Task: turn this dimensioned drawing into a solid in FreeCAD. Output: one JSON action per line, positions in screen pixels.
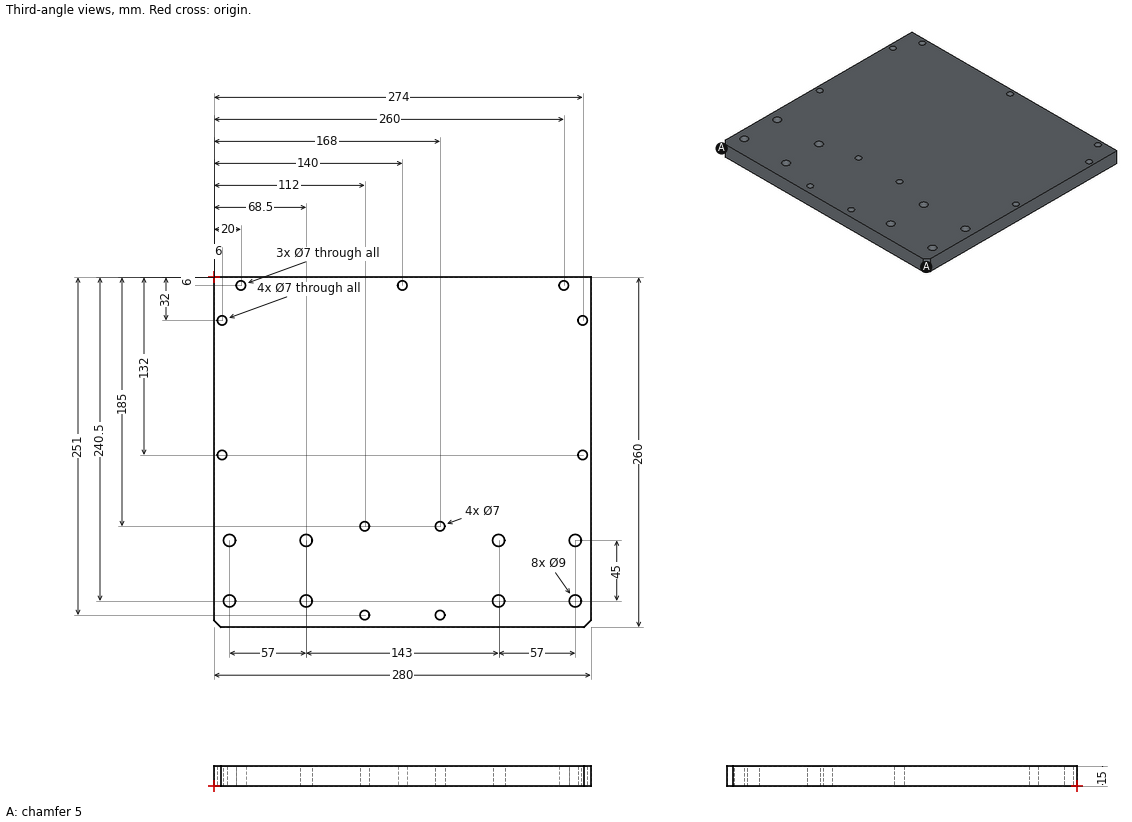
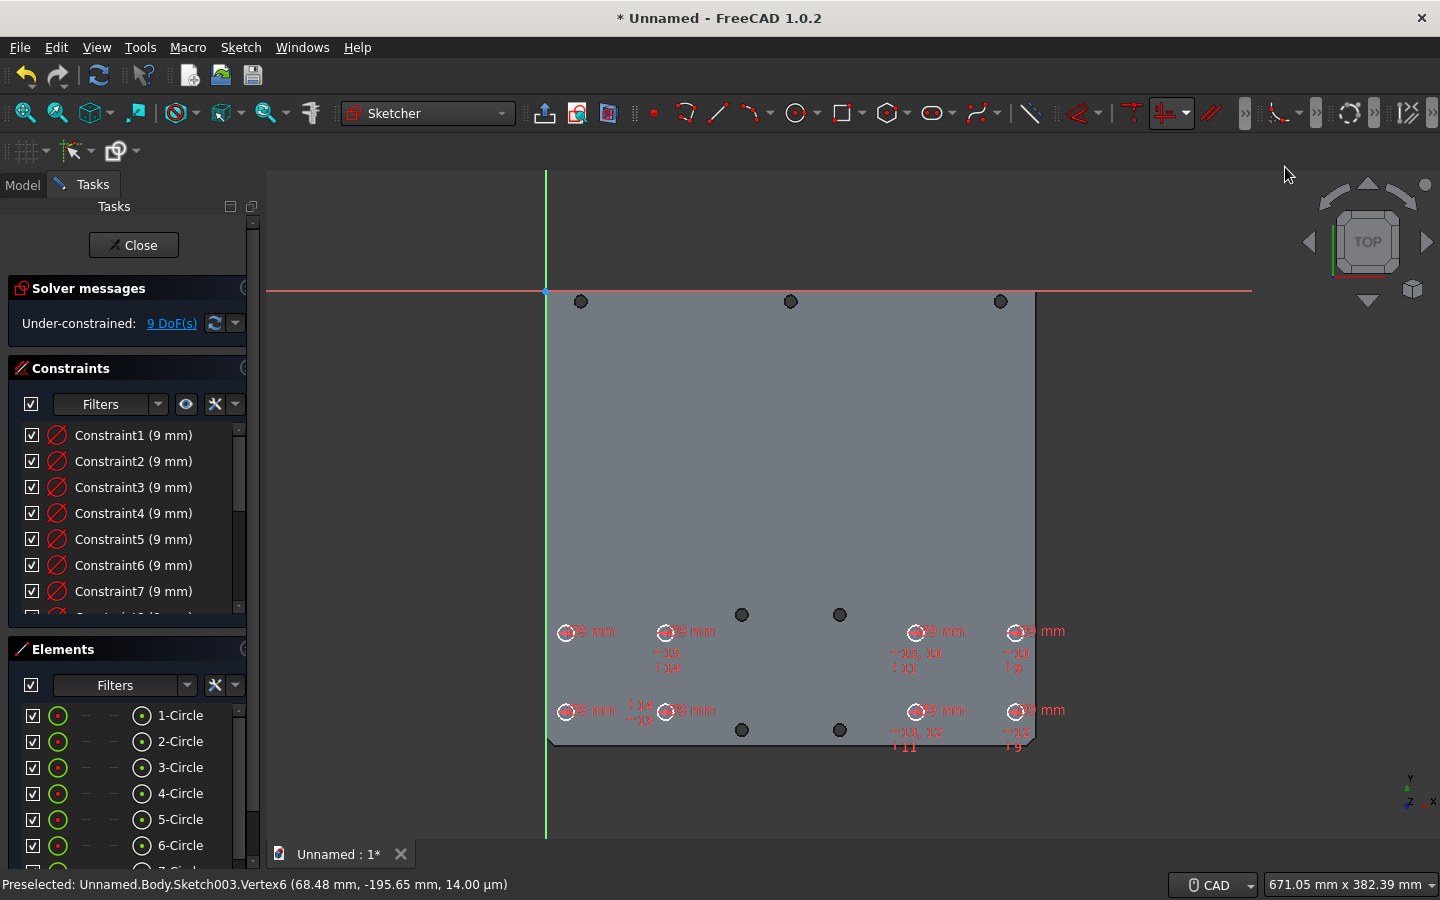
{"action": "left_click", "coordinate": [666, 633]}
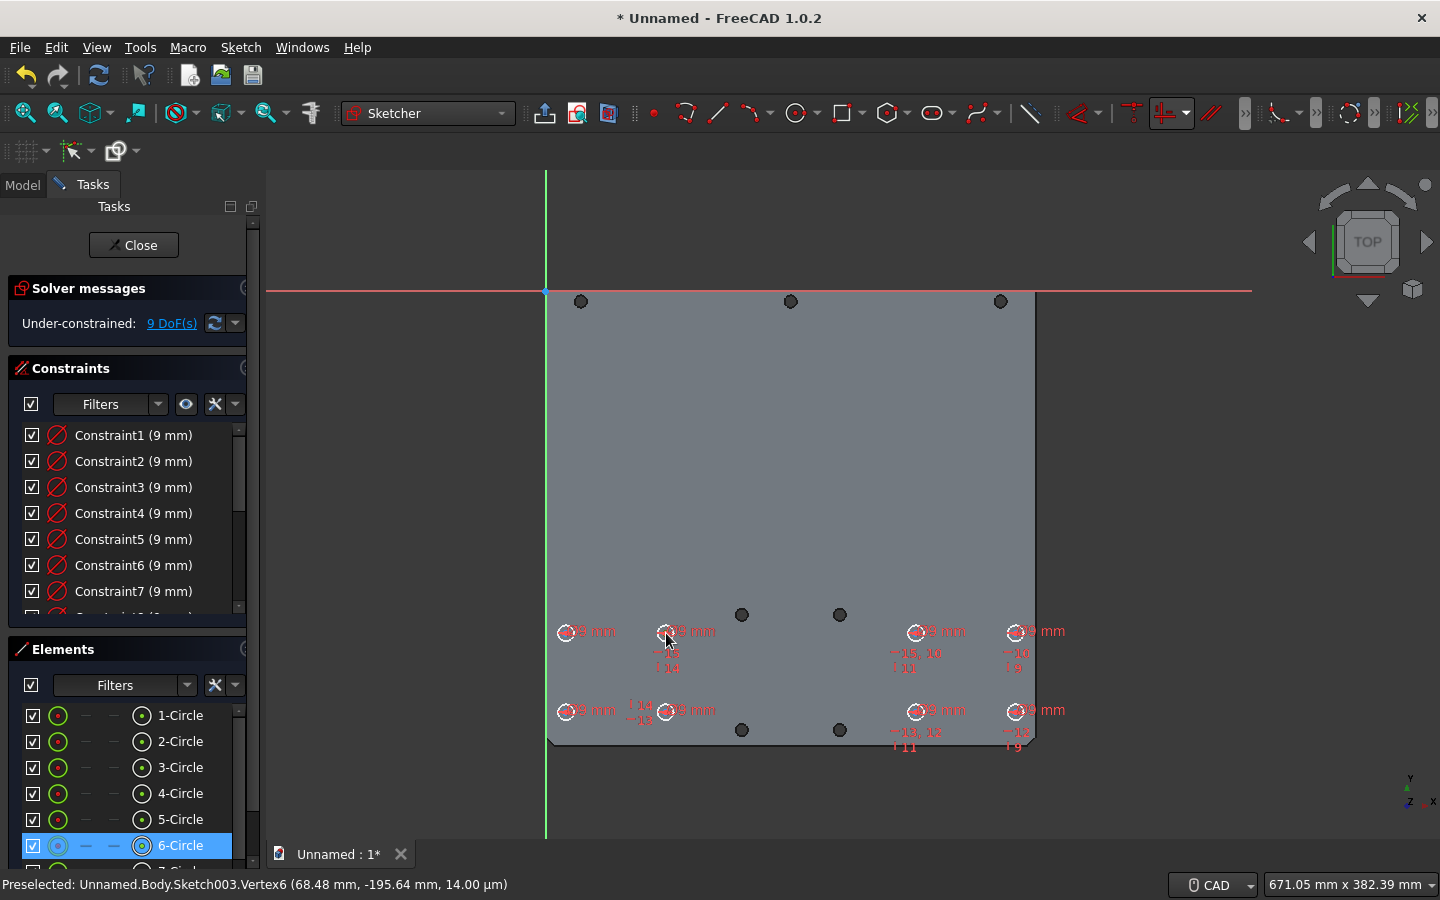
{"action": "left_click", "coordinate": [566, 633]}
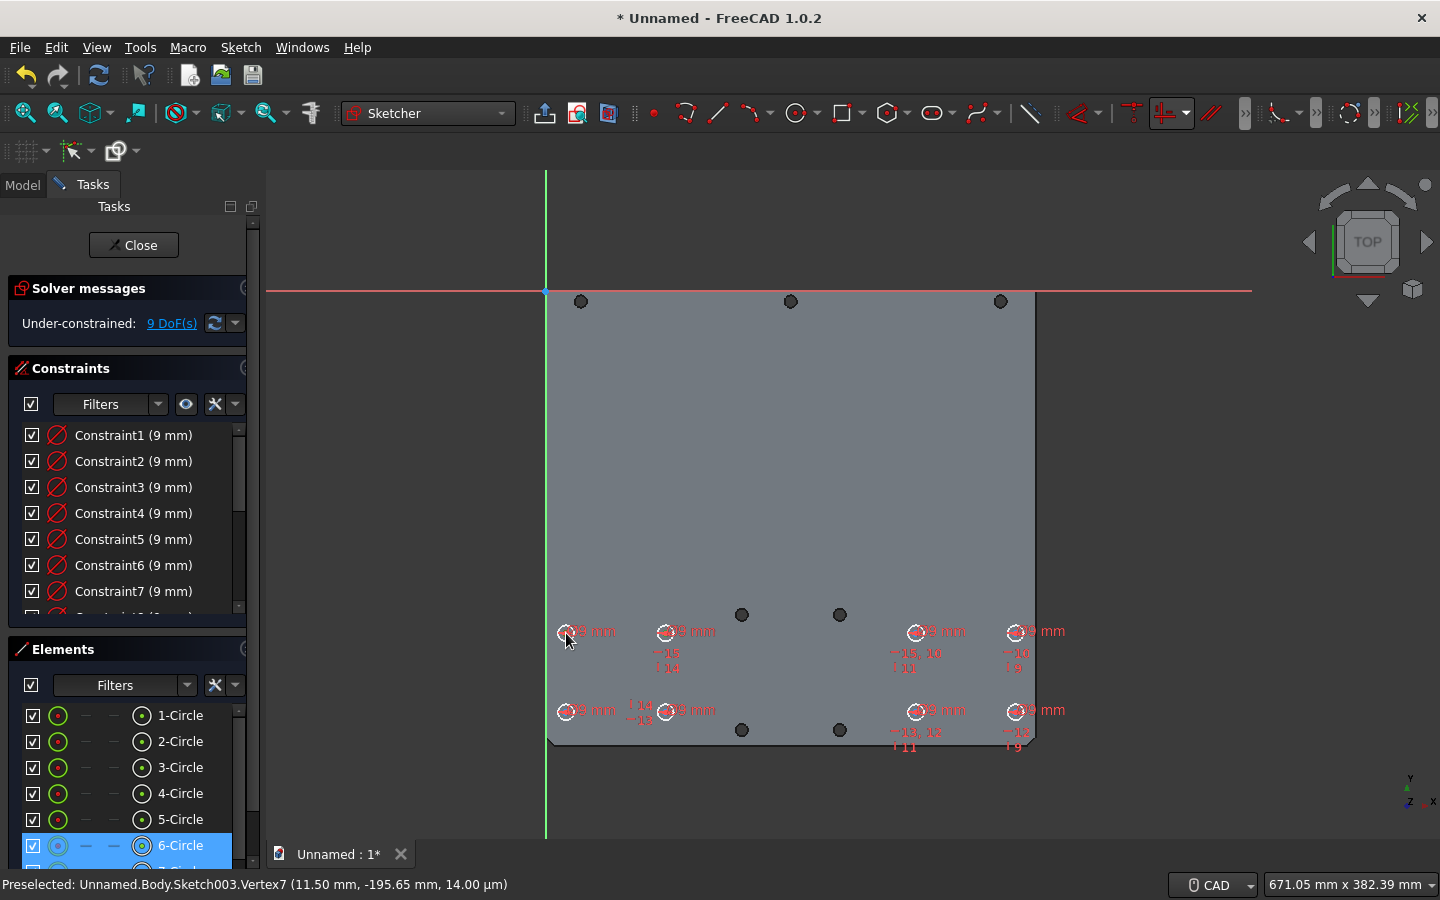
{"action": "key", "text": "h"}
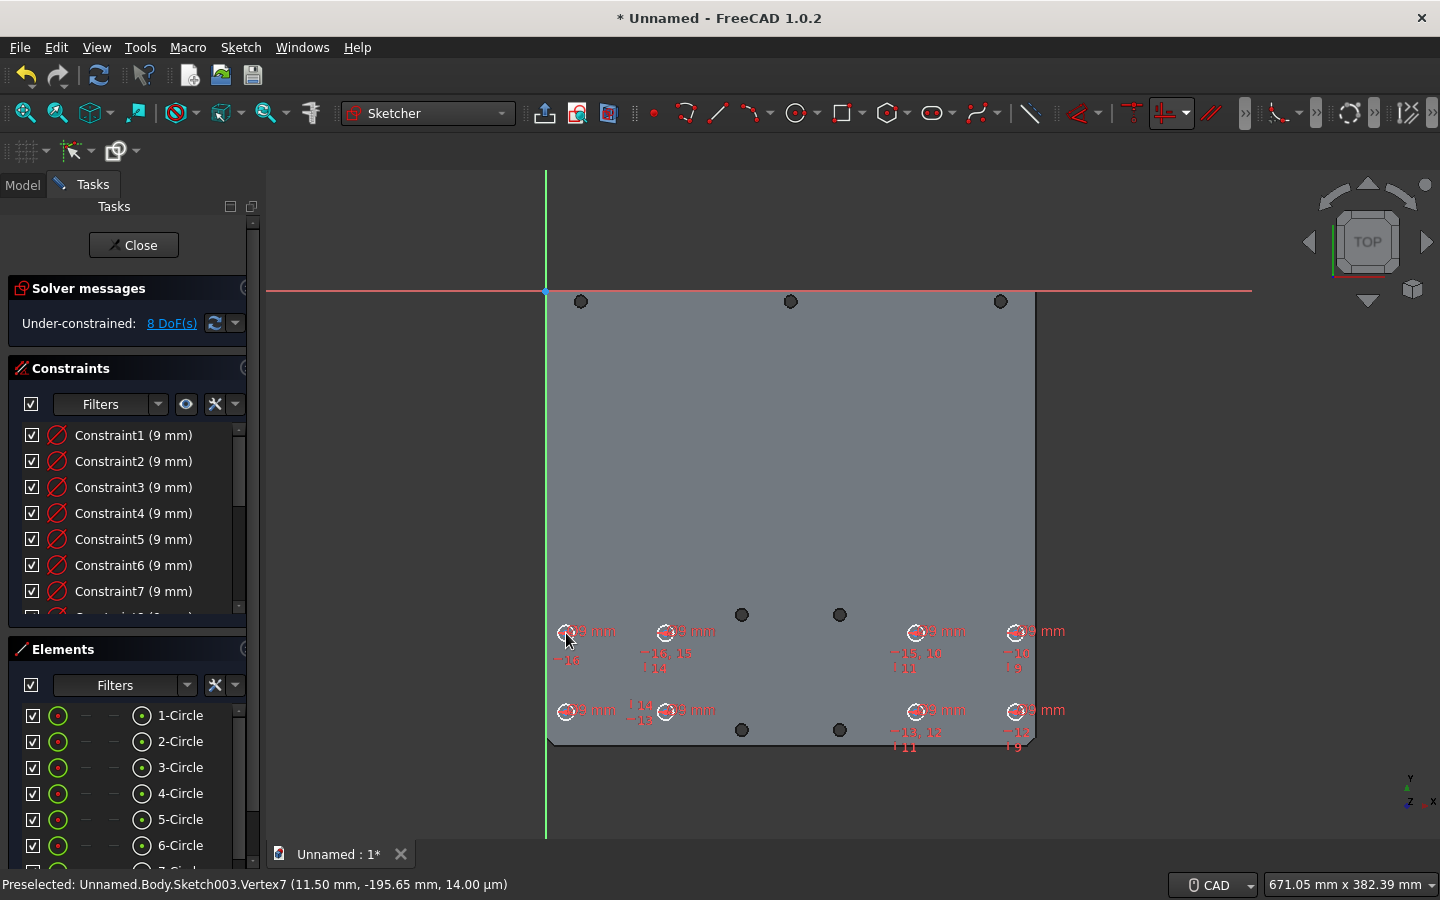
{"action": "left_click", "coordinate": [566, 633]}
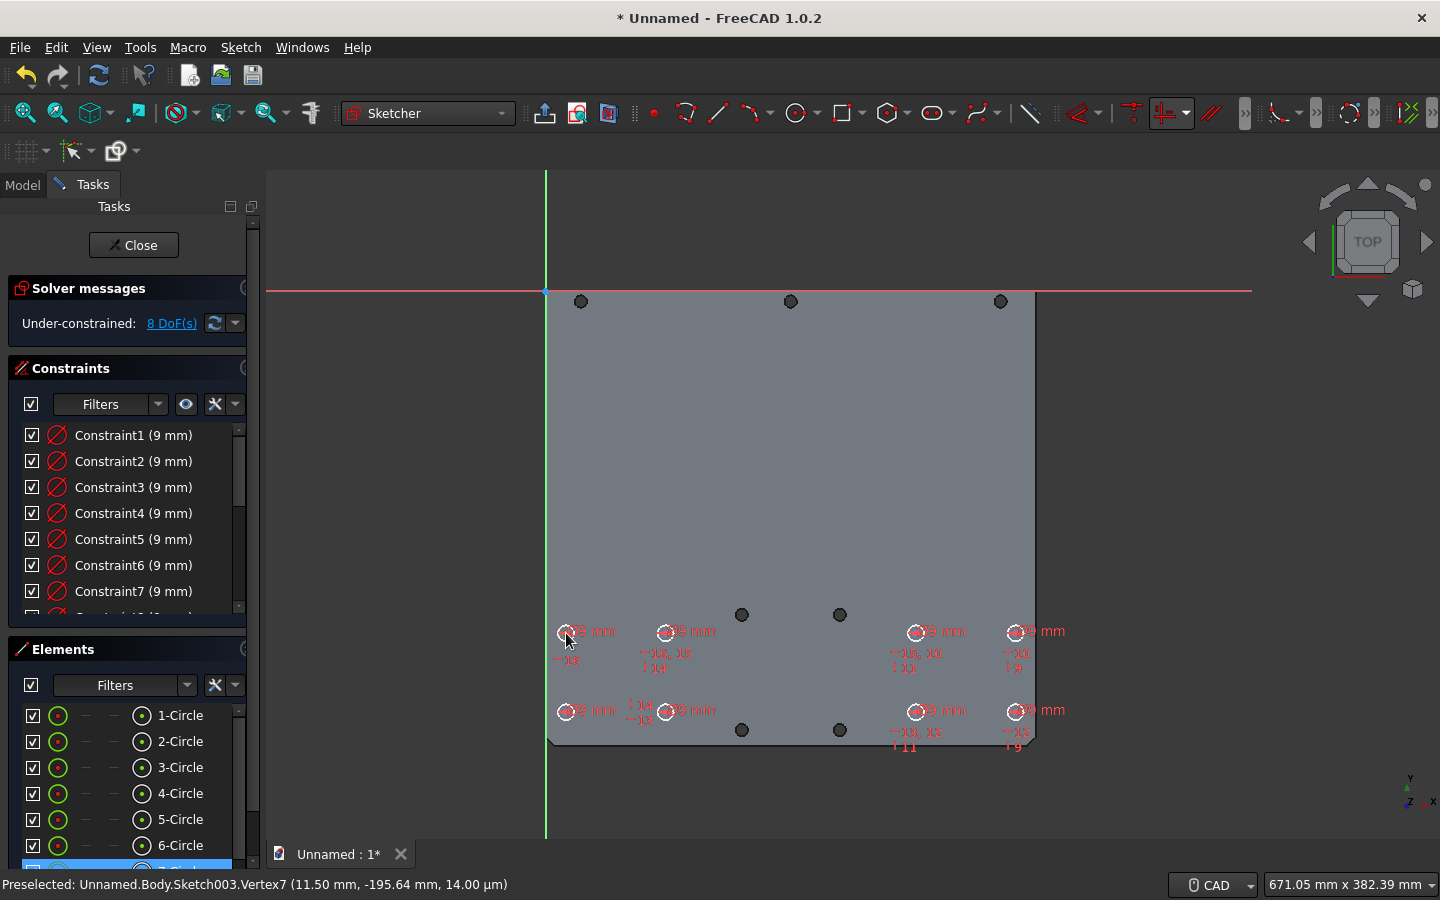
{"action": "left_click", "coordinate": [566, 712]}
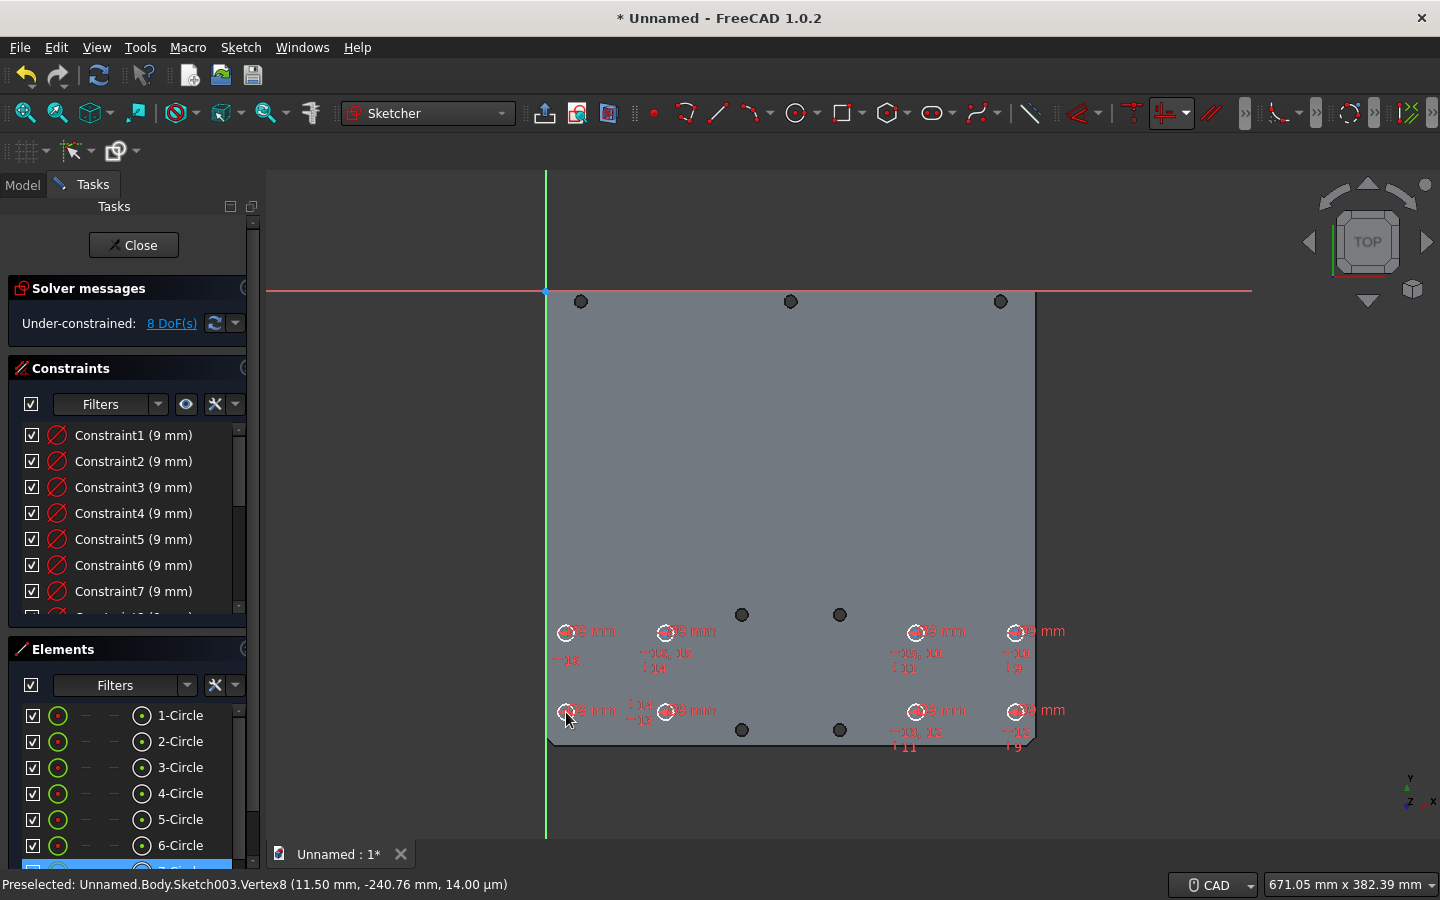
{"action": "left_click", "coordinate": [1188, 114]}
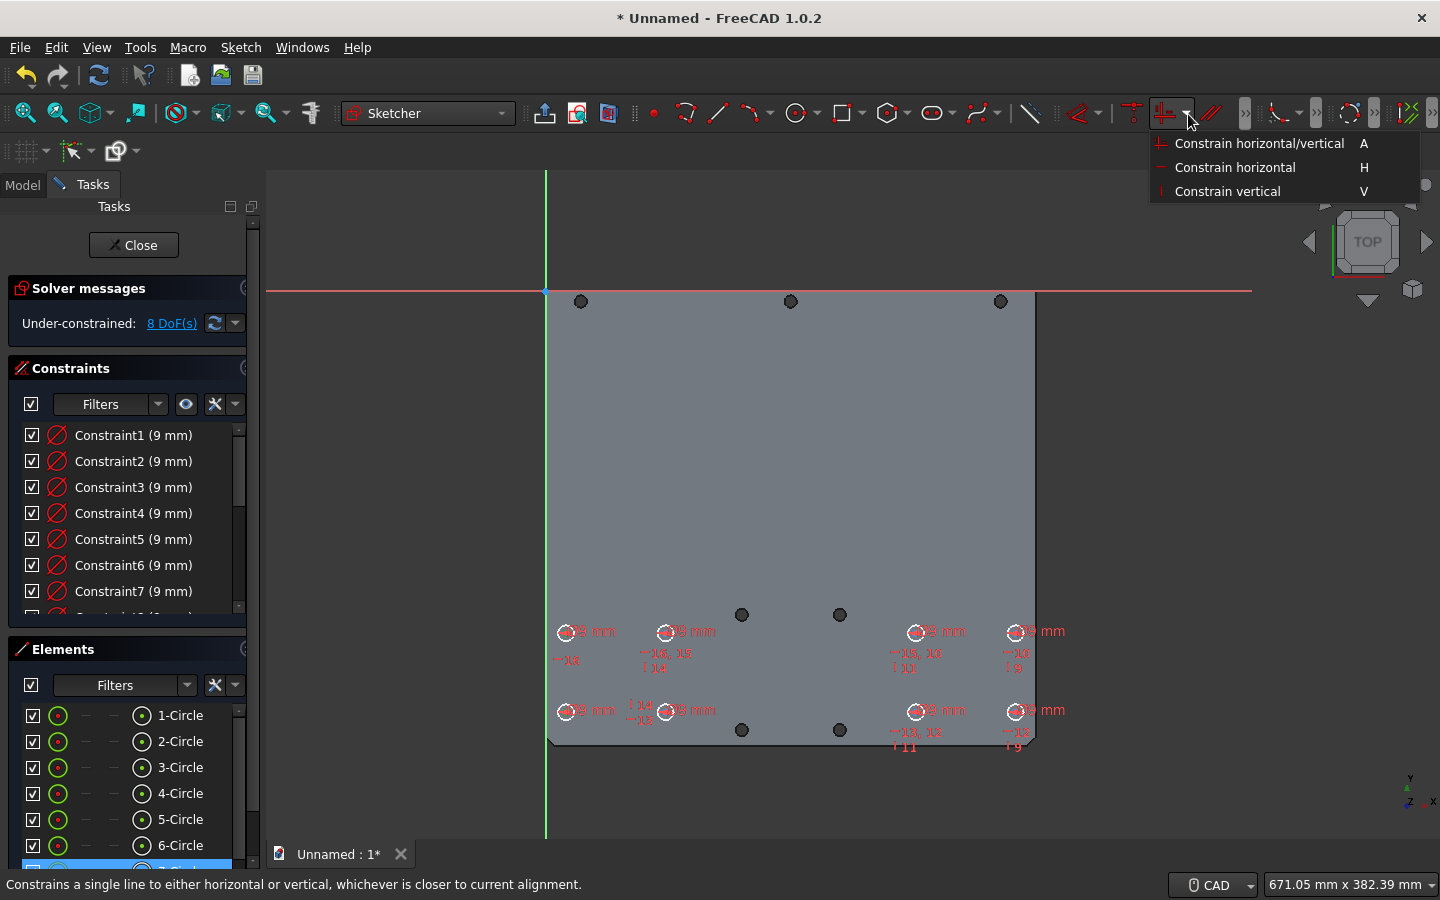
{"action": "left_click", "coordinate": [1285, 191]}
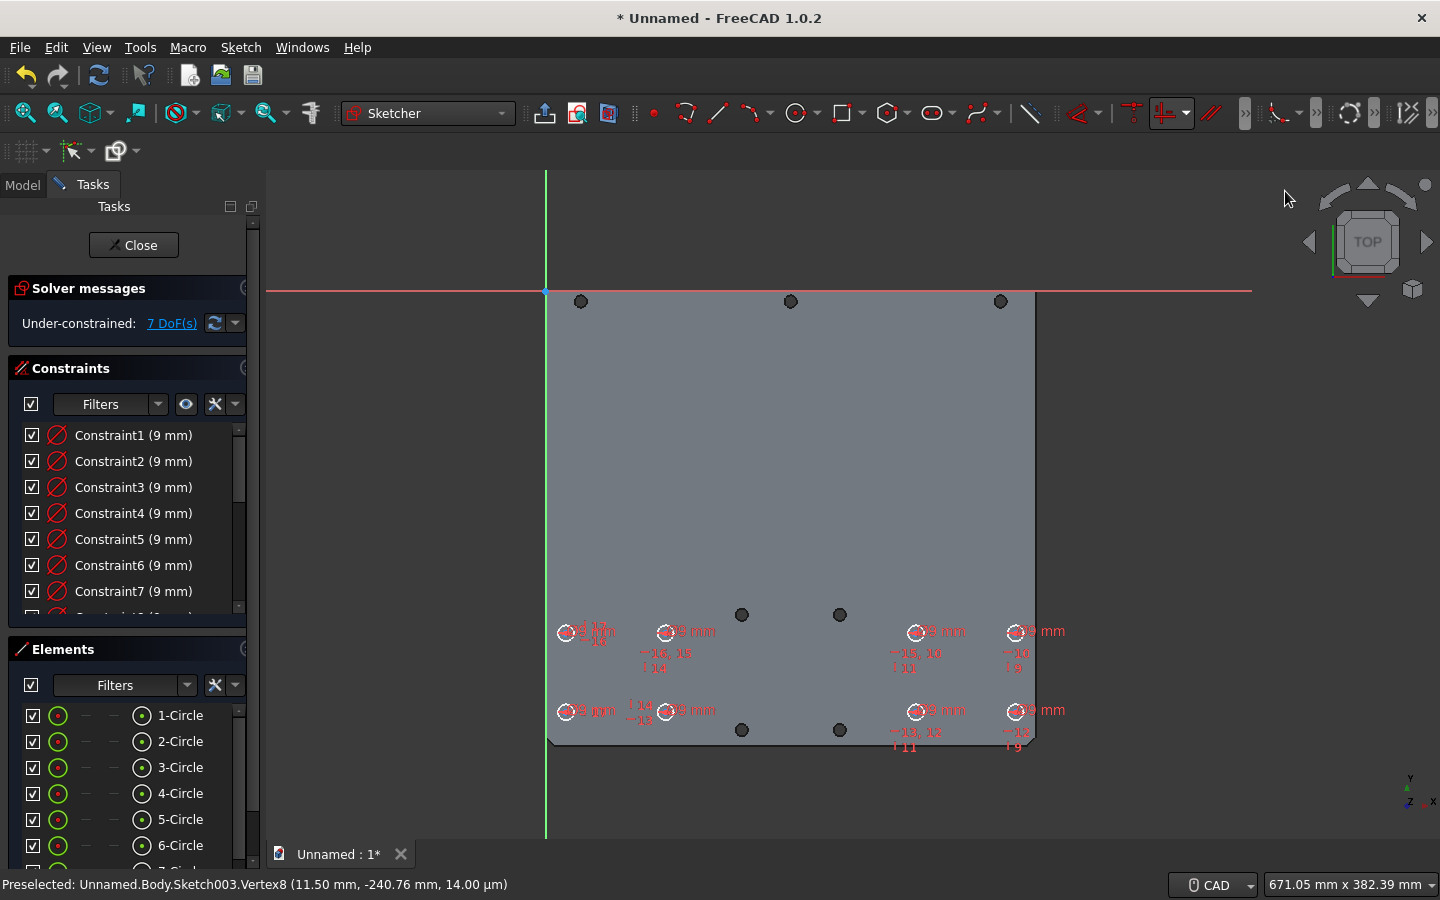
{"action": "left_click", "coordinate": [666, 712]}